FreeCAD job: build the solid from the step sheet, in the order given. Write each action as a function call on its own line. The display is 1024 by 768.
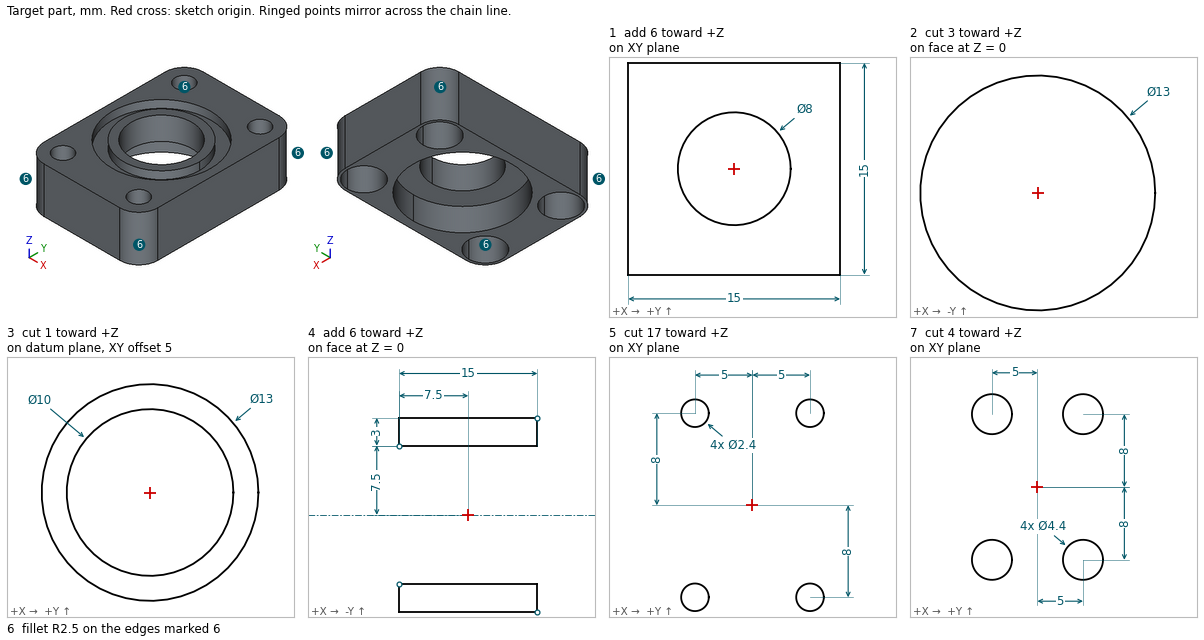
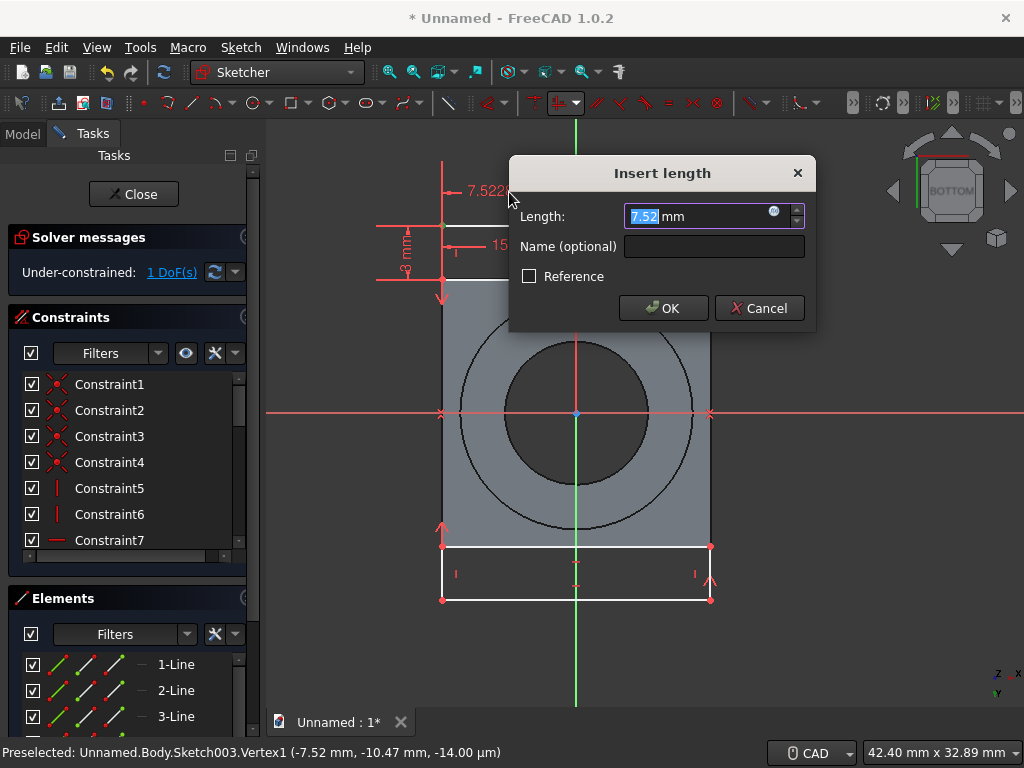
text(7.5)
key(Return)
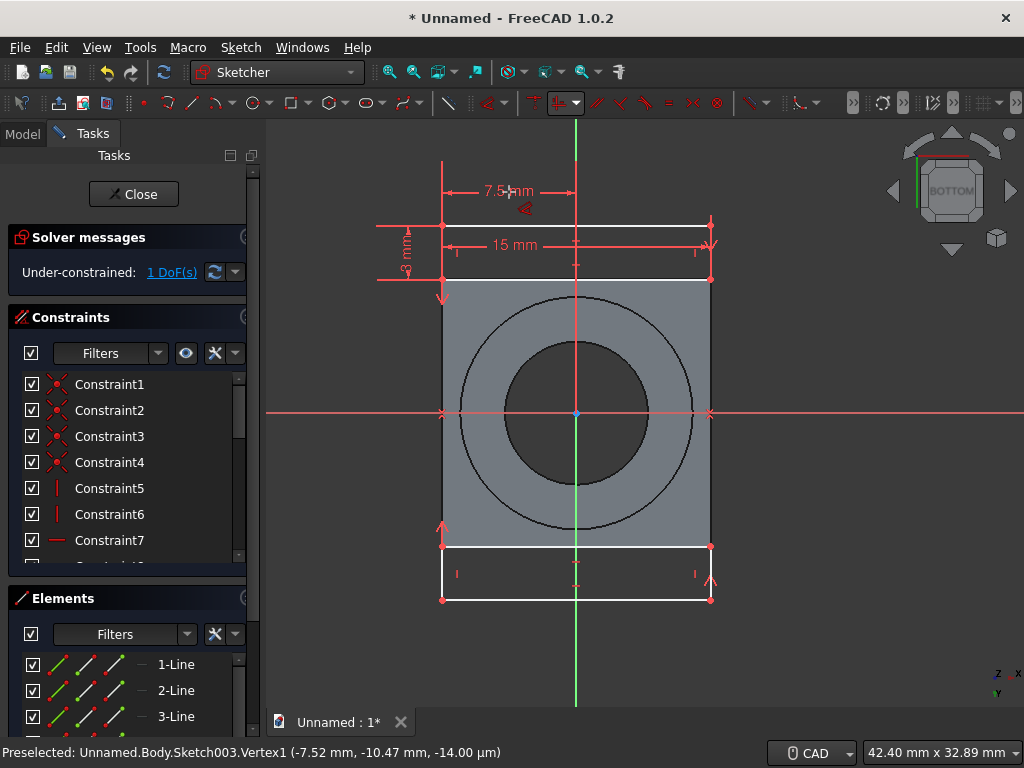
click(442, 280)
click(408, 346)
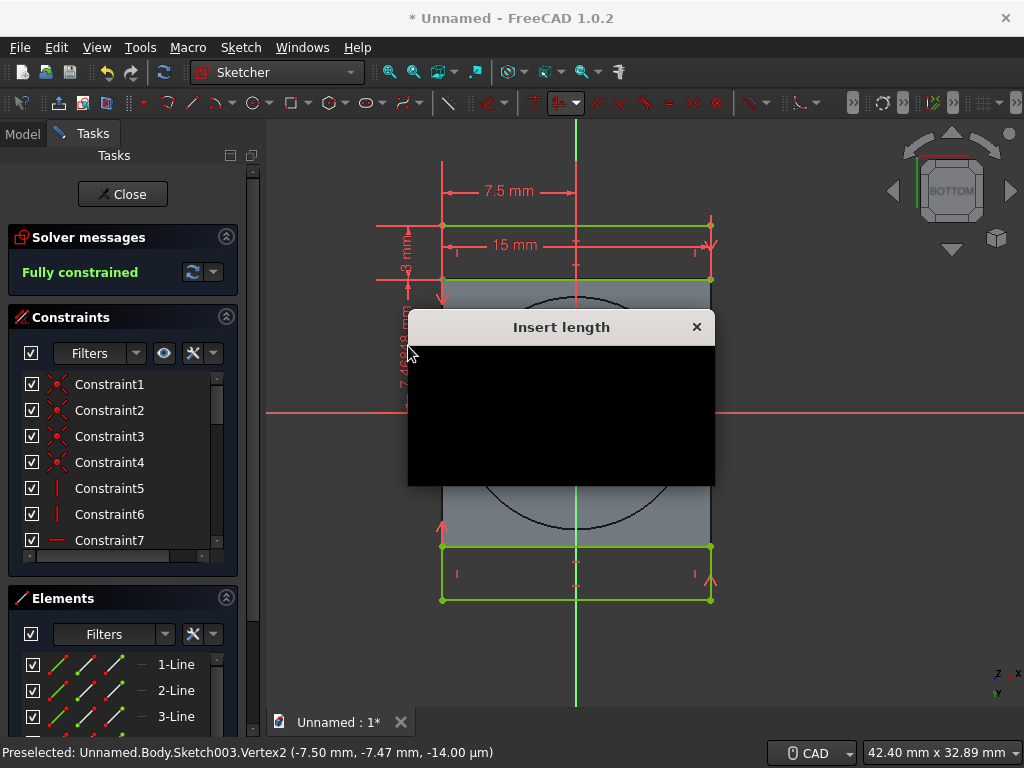
text(7.5)
key(Return)
key(Escape)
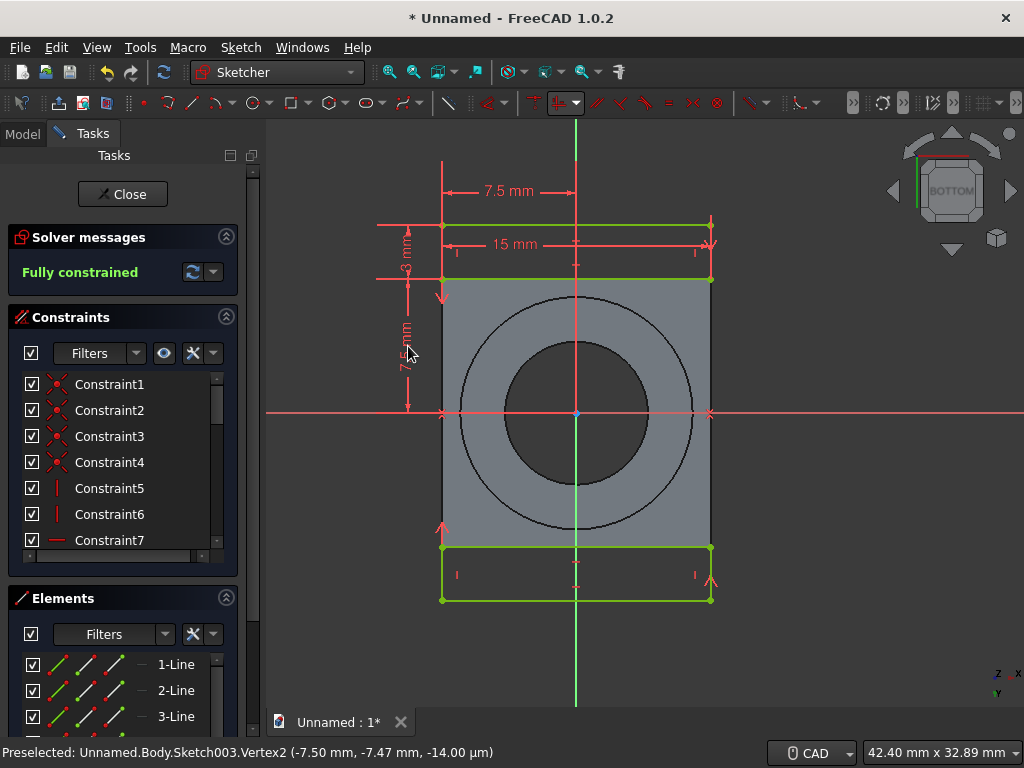
click(123, 194)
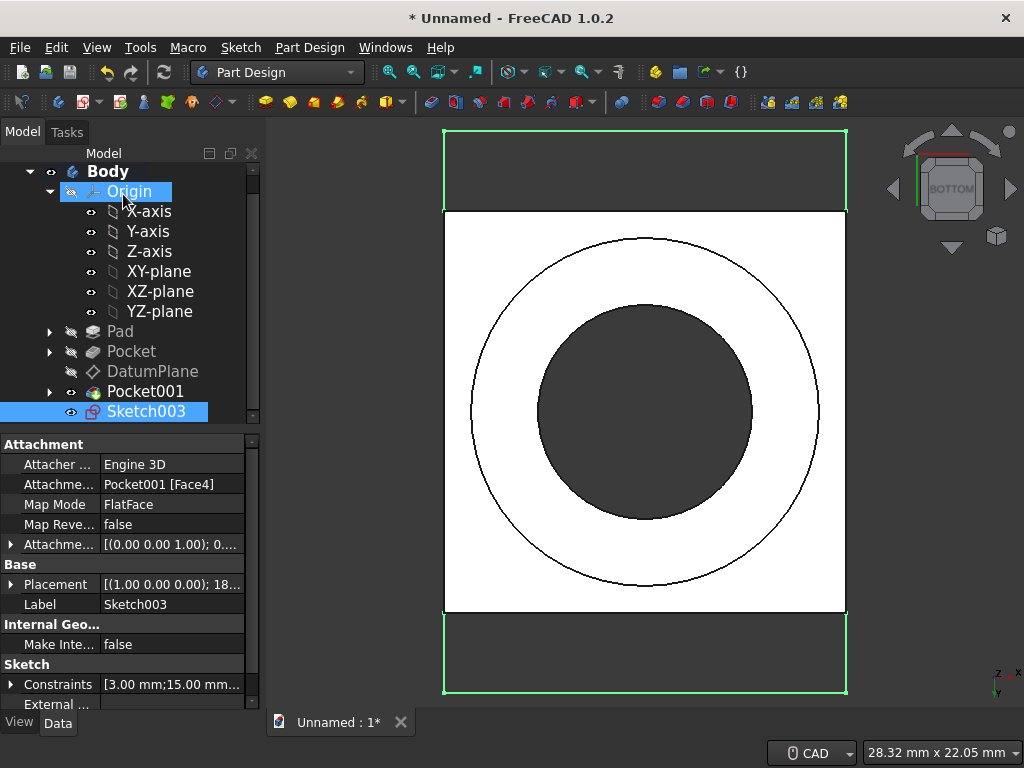
click(266, 102)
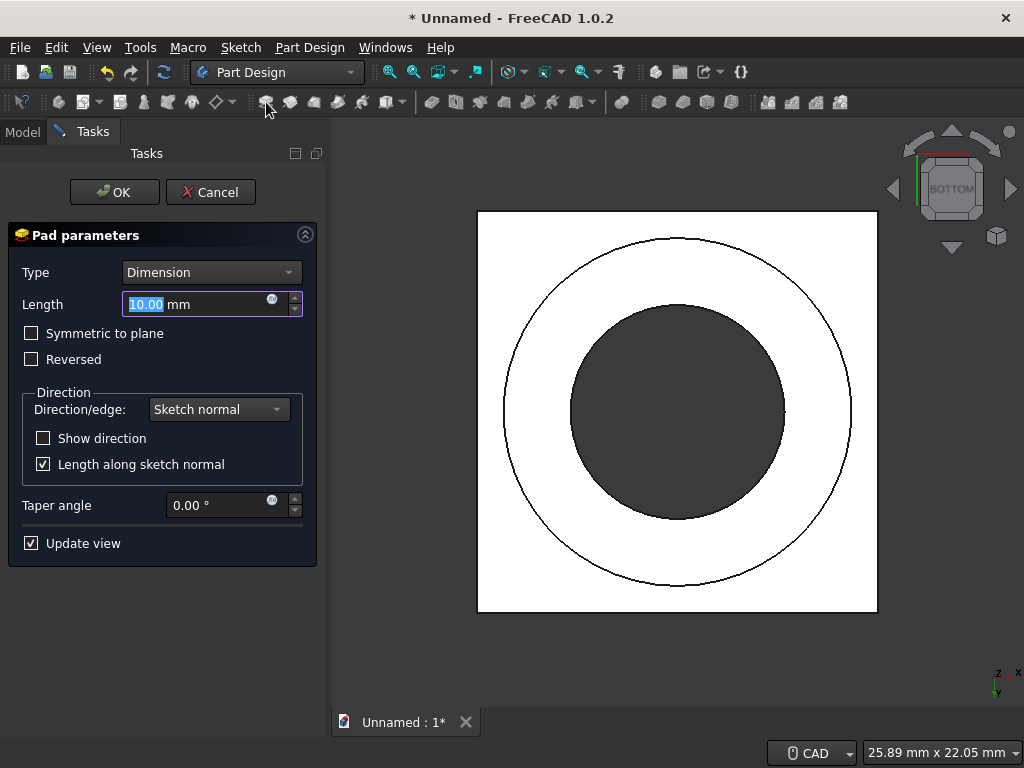
text(6)
key(Tab)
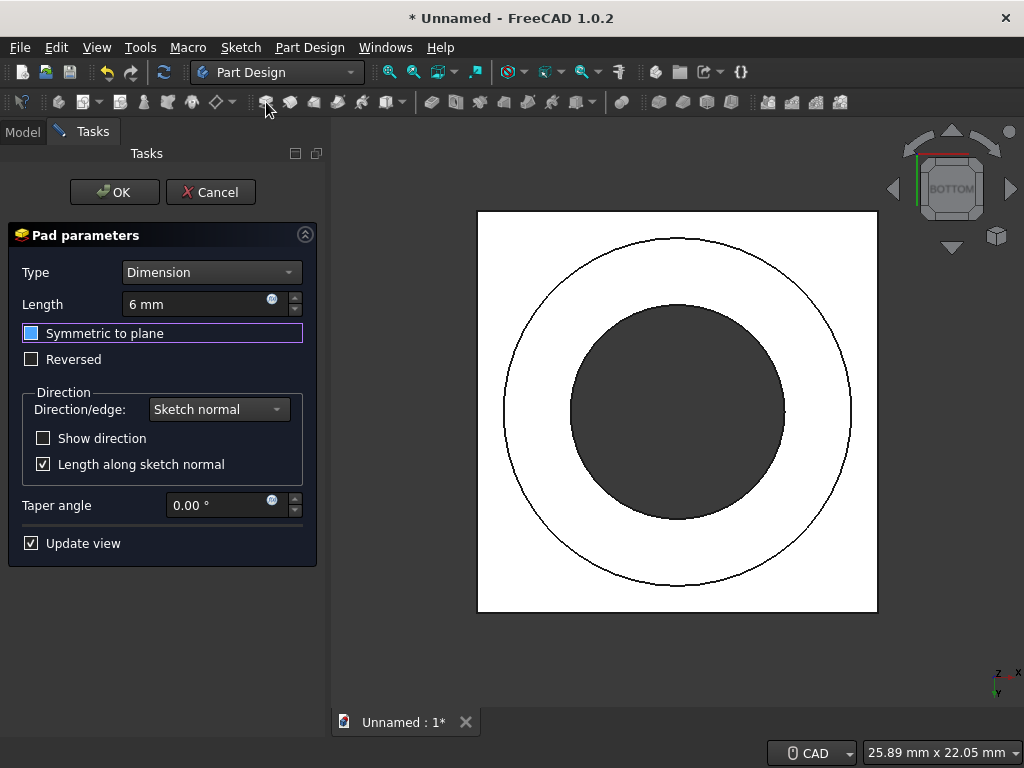
click(30, 359)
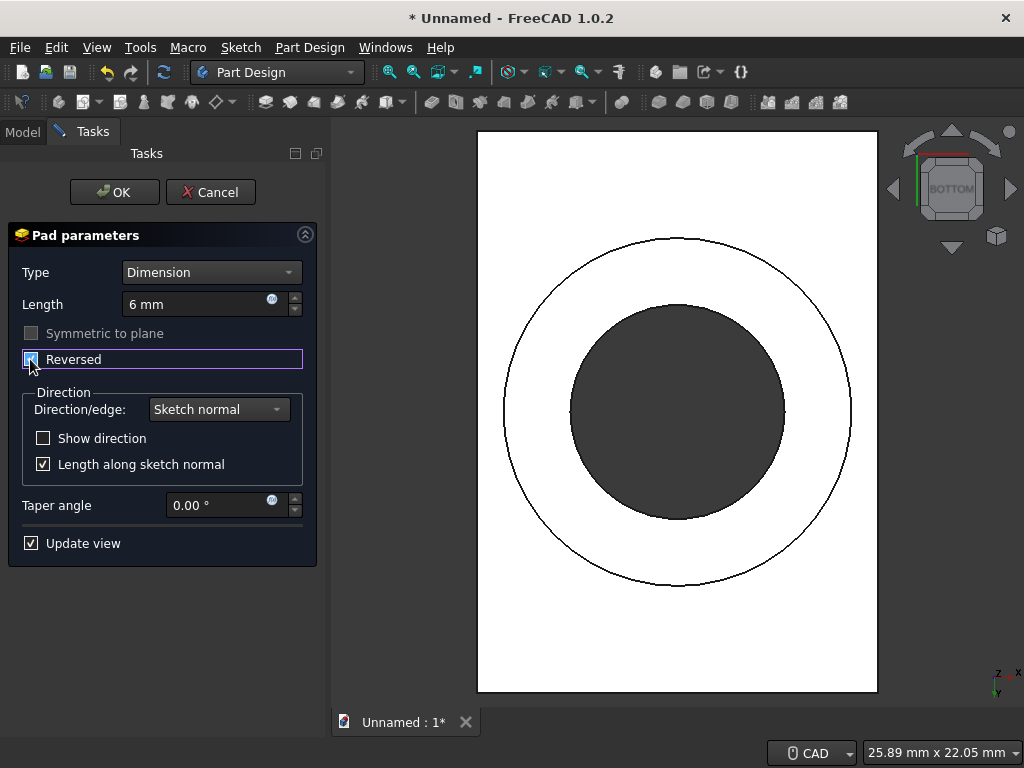
click(115, 192)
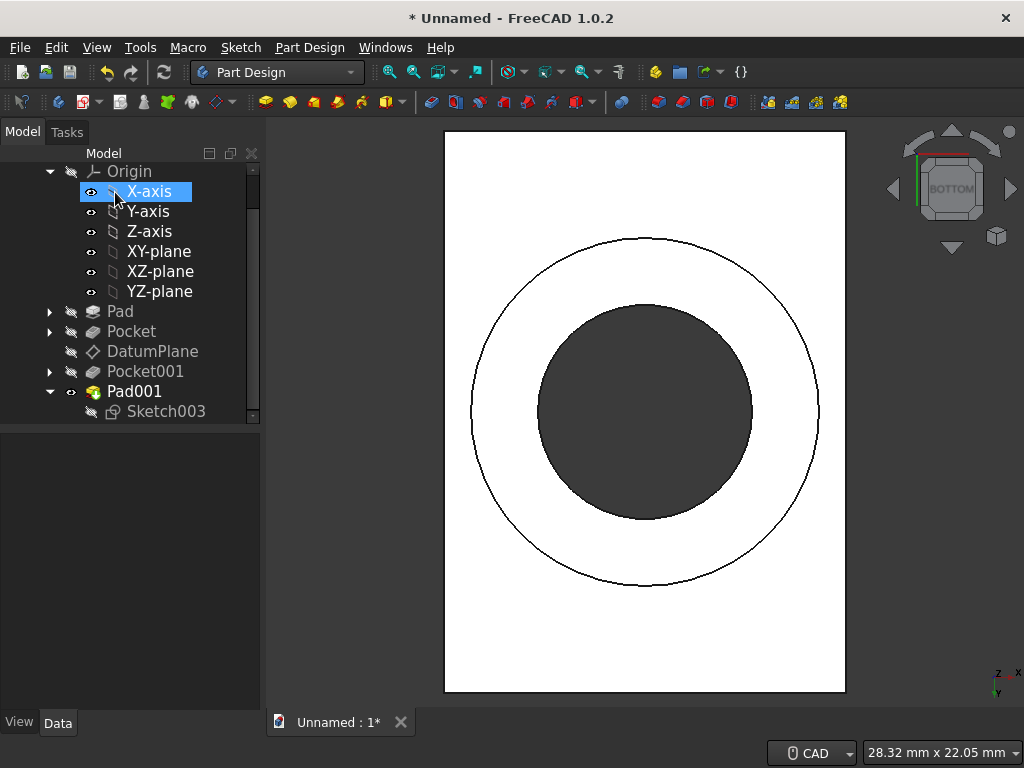
click(84, 102)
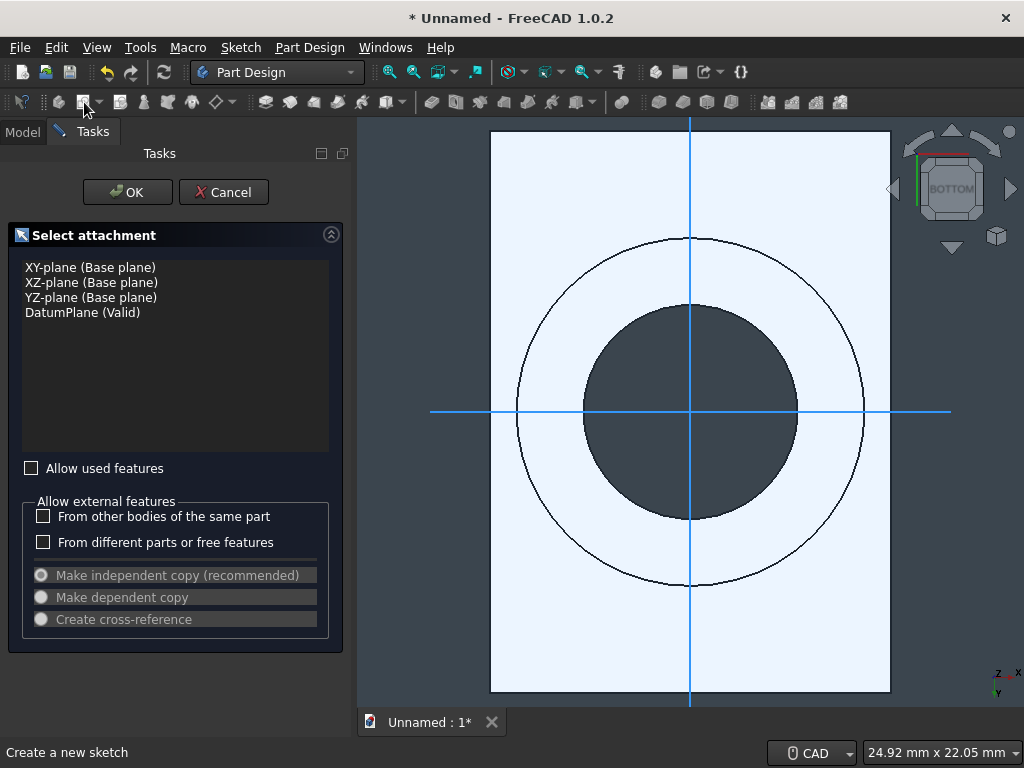
click(82, 268)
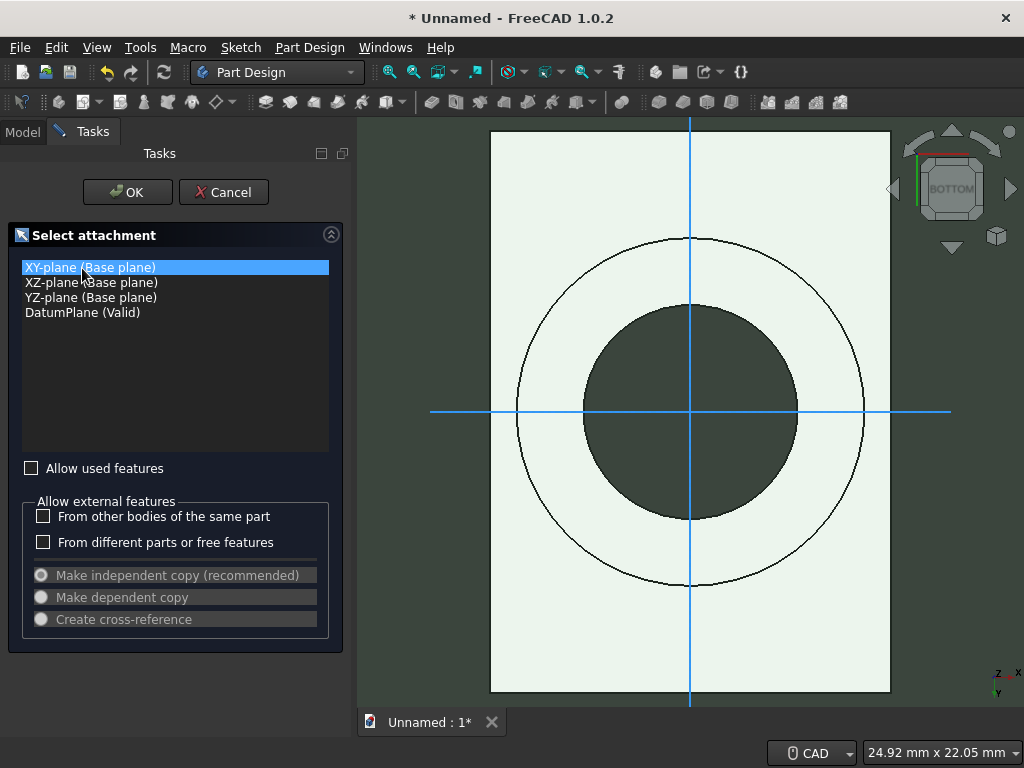
click(128, 192)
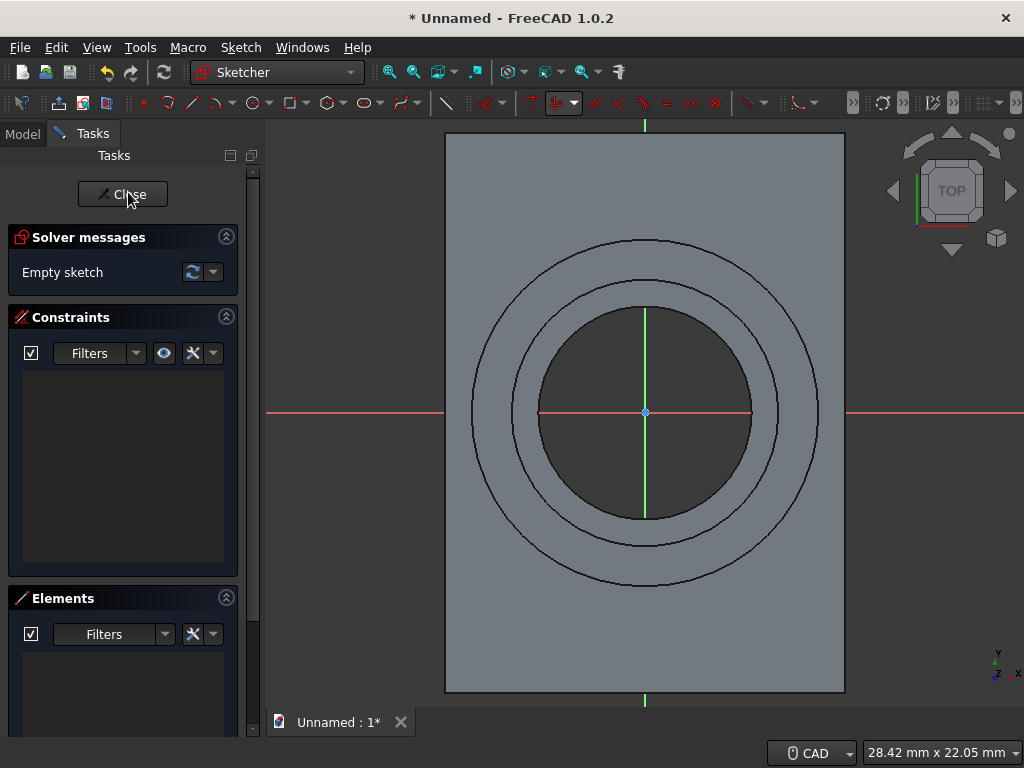
click(108, 104)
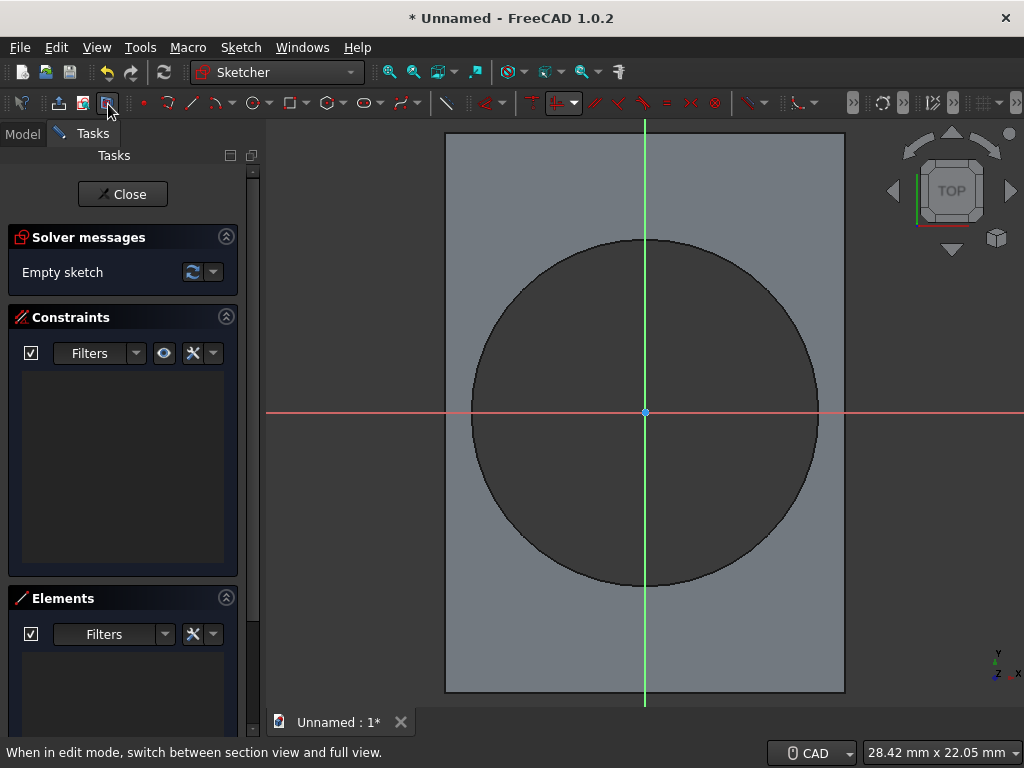
scroll(294, 413, down, 1)